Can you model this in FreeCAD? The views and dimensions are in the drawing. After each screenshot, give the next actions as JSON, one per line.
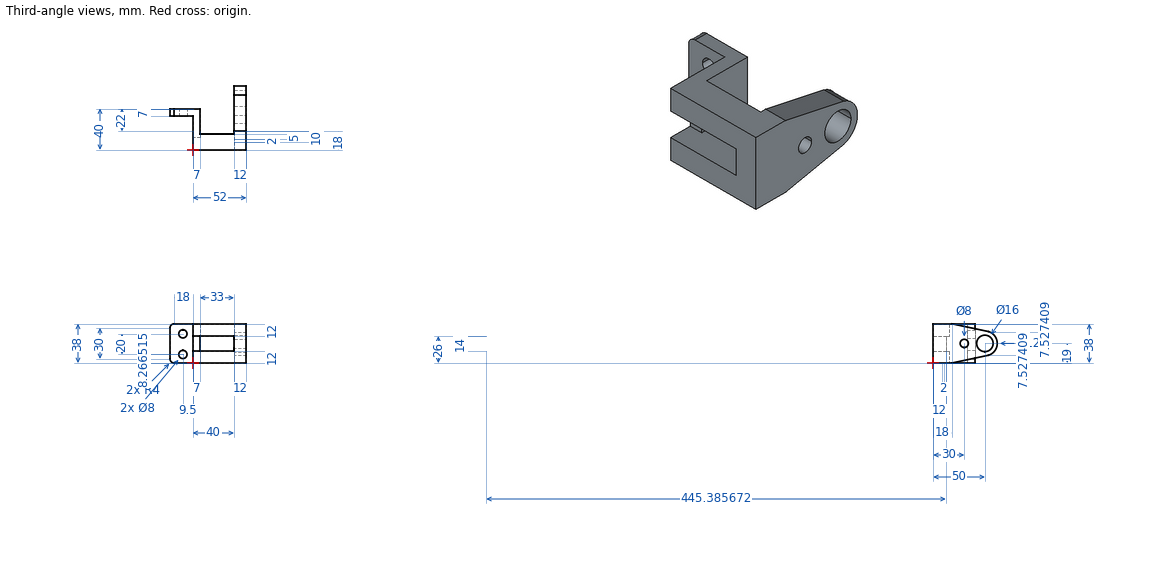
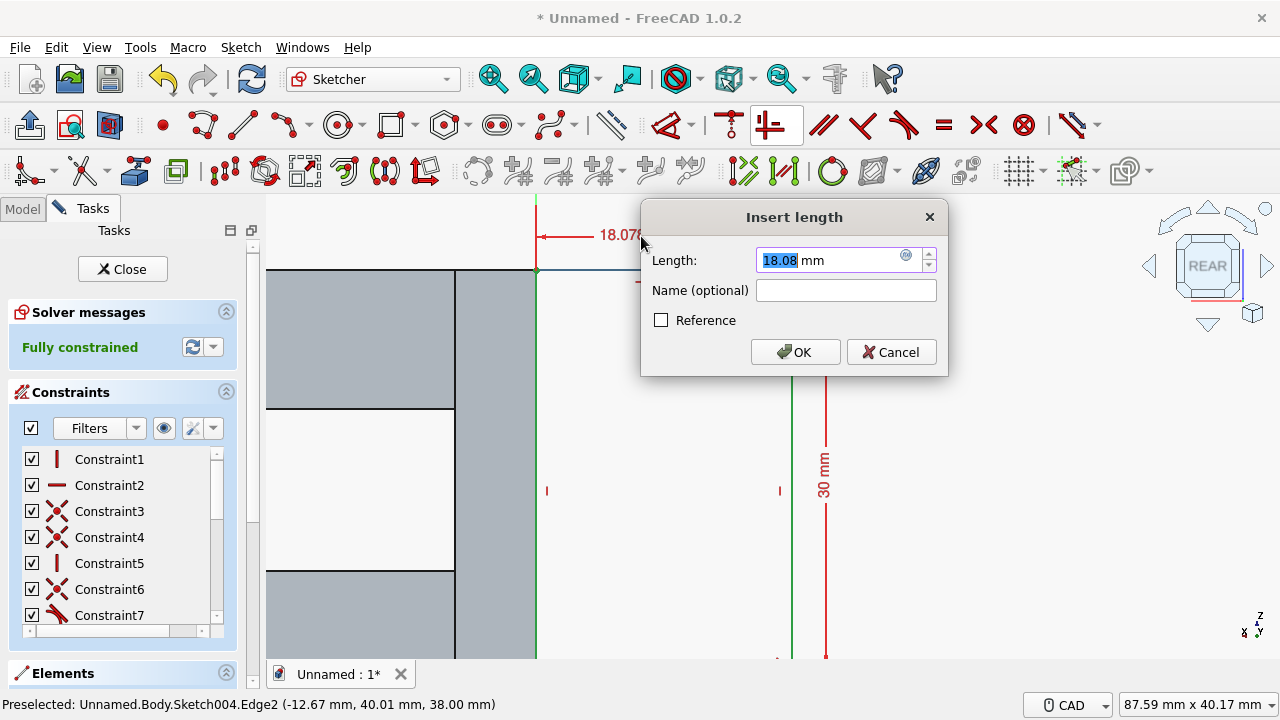
{"action": "type", "text": "18"}
{"action": "key", "text": "Return"}
{"action": "key", "text": "Escape"}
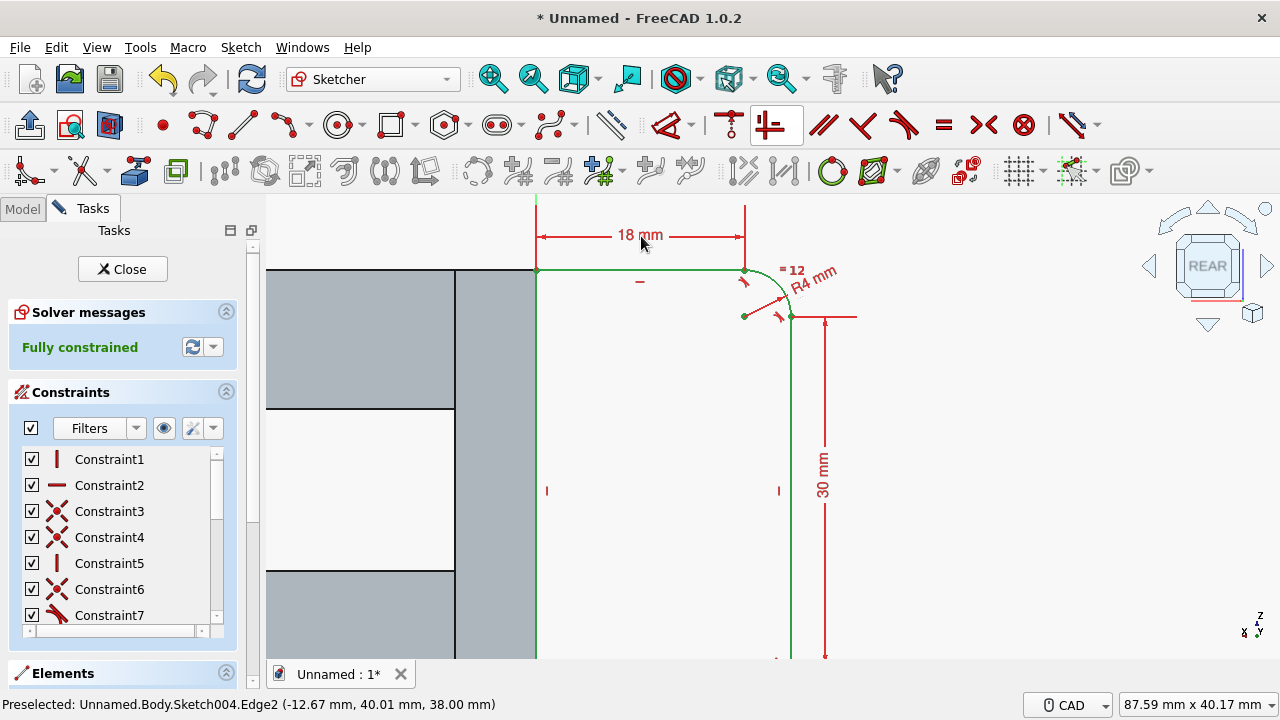
{"action": "left_click", "coordinate": [123, 269]}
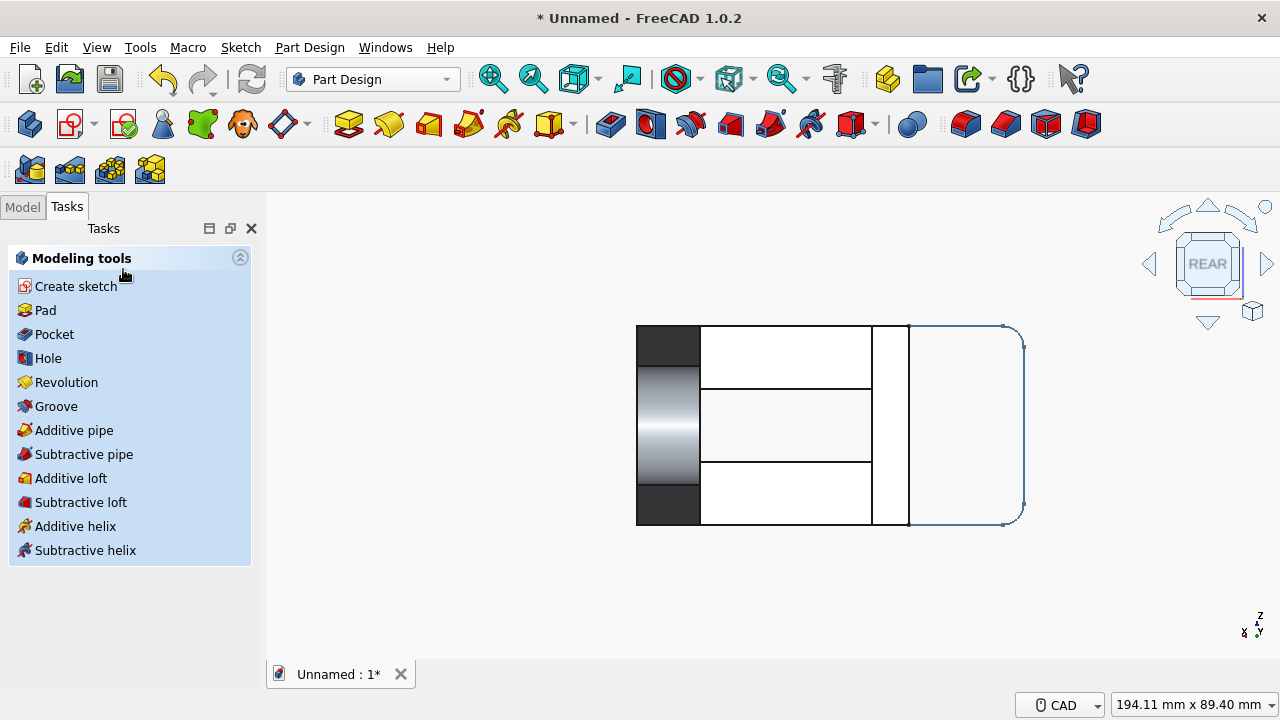
{"action": "left_click", "coordinate": [350, 124]}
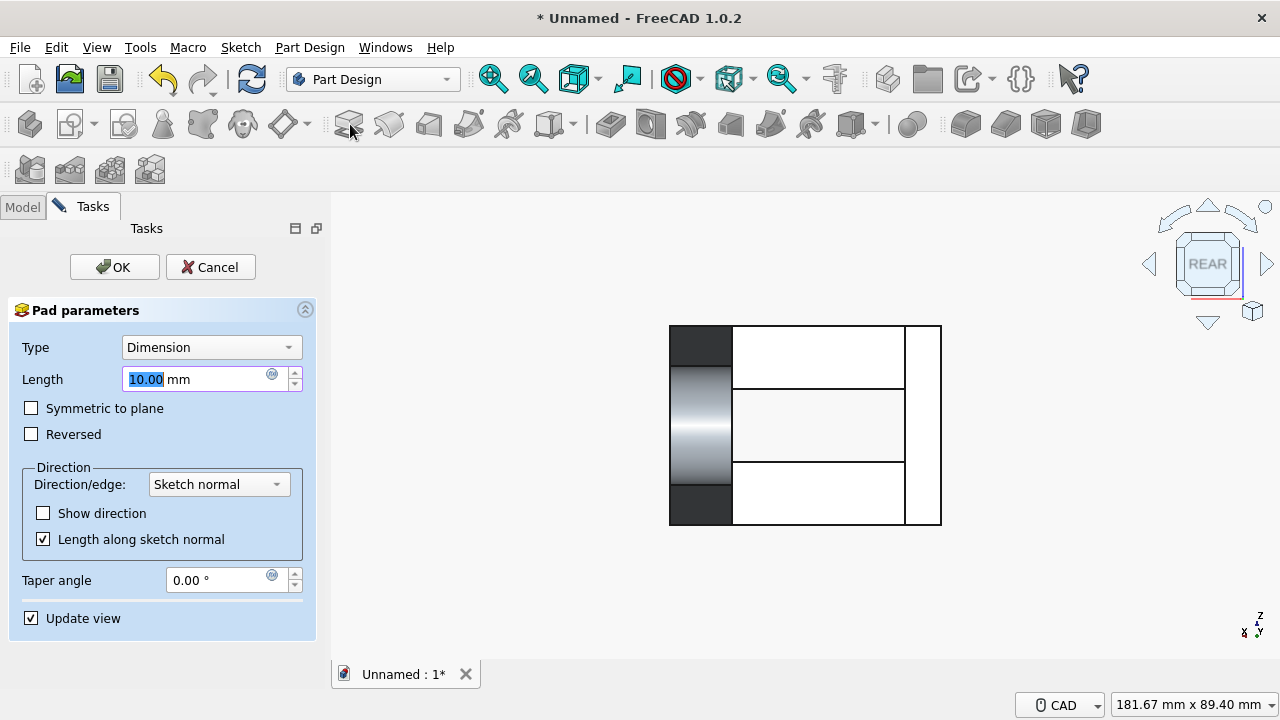
{"action": "type", "text": "7"}
{"action": "key", "text": "Tab"}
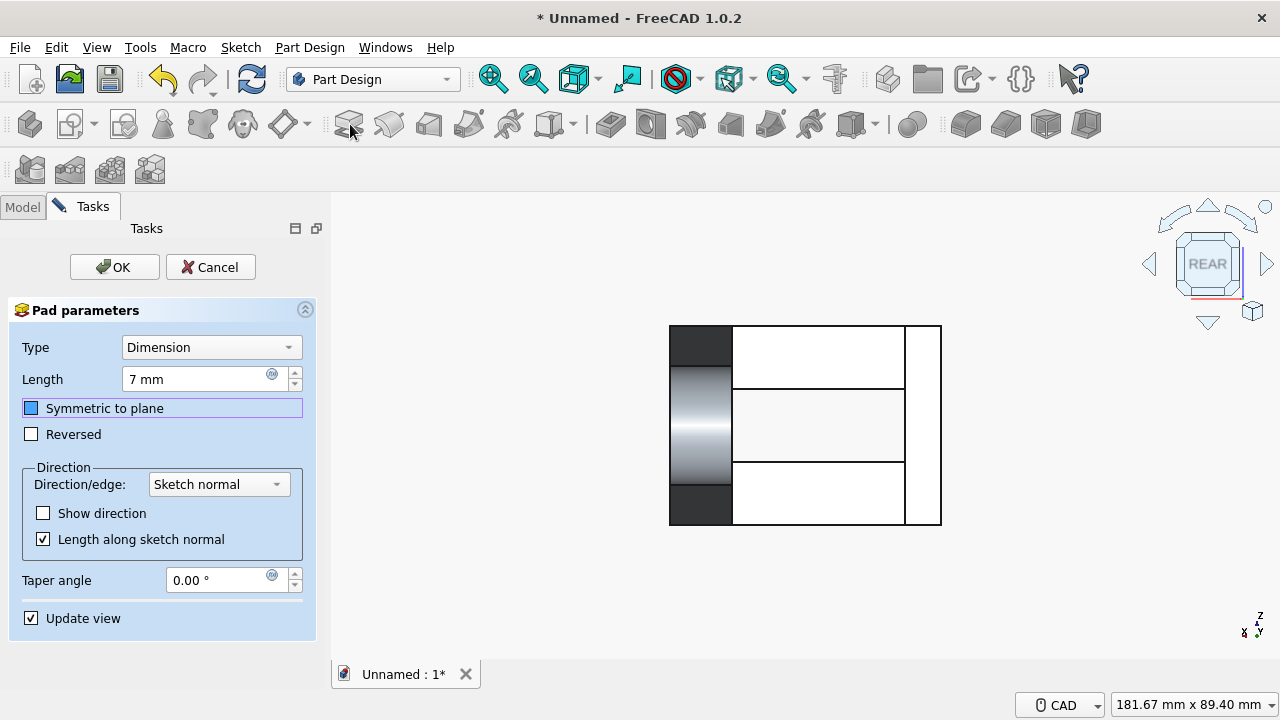
{"action": "left_click", "coordinate": [30, 434]}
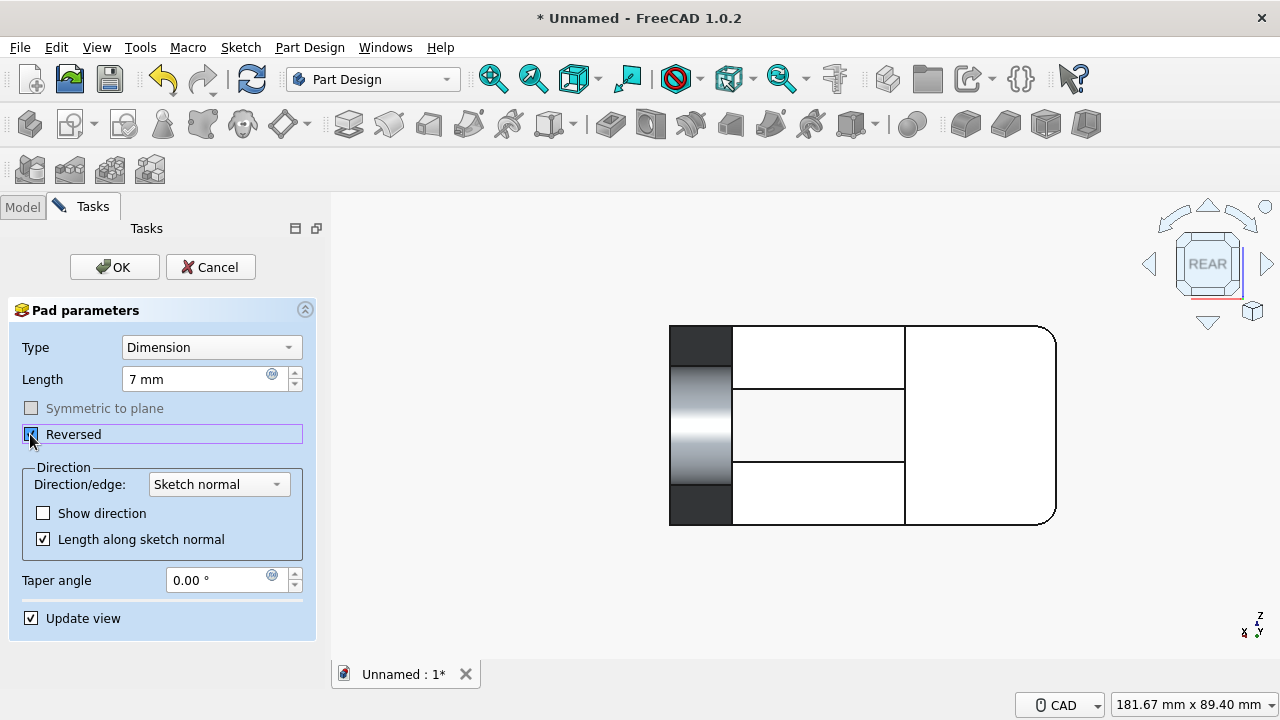
{"action": "left_click", "coordinate": [115, 267]}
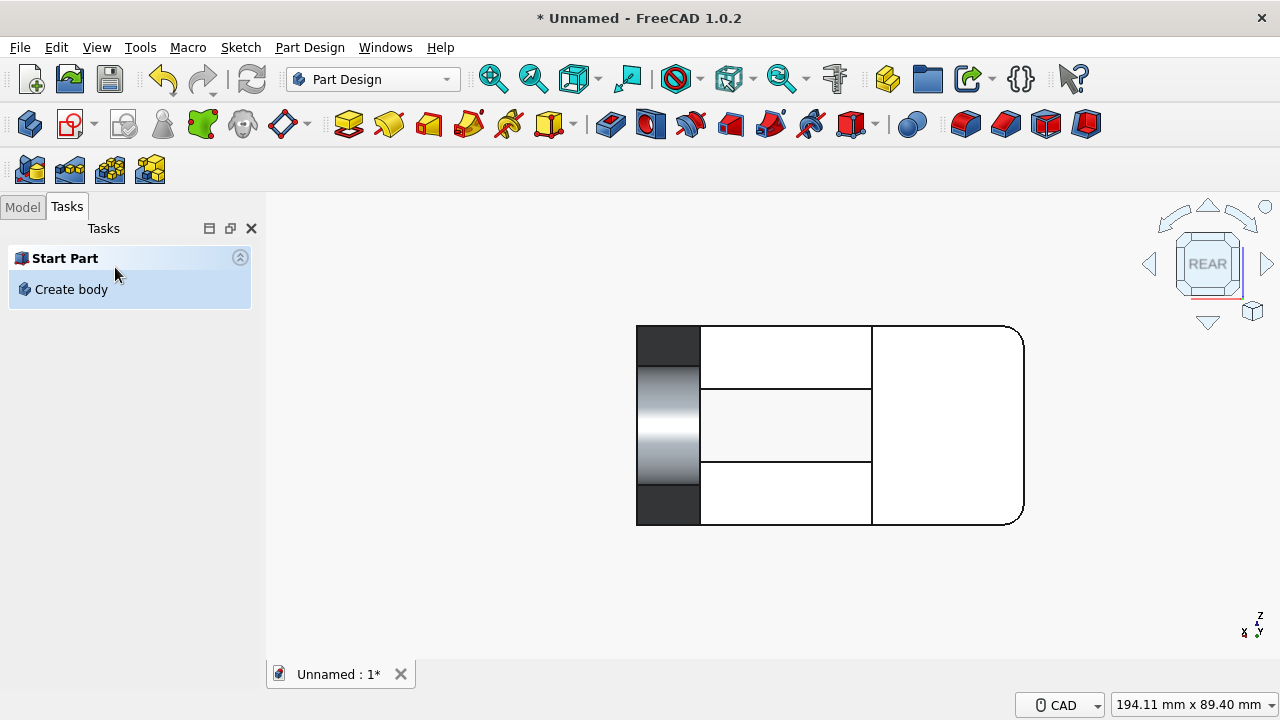
{"action": "left_click", "coordinate": [494, 80]}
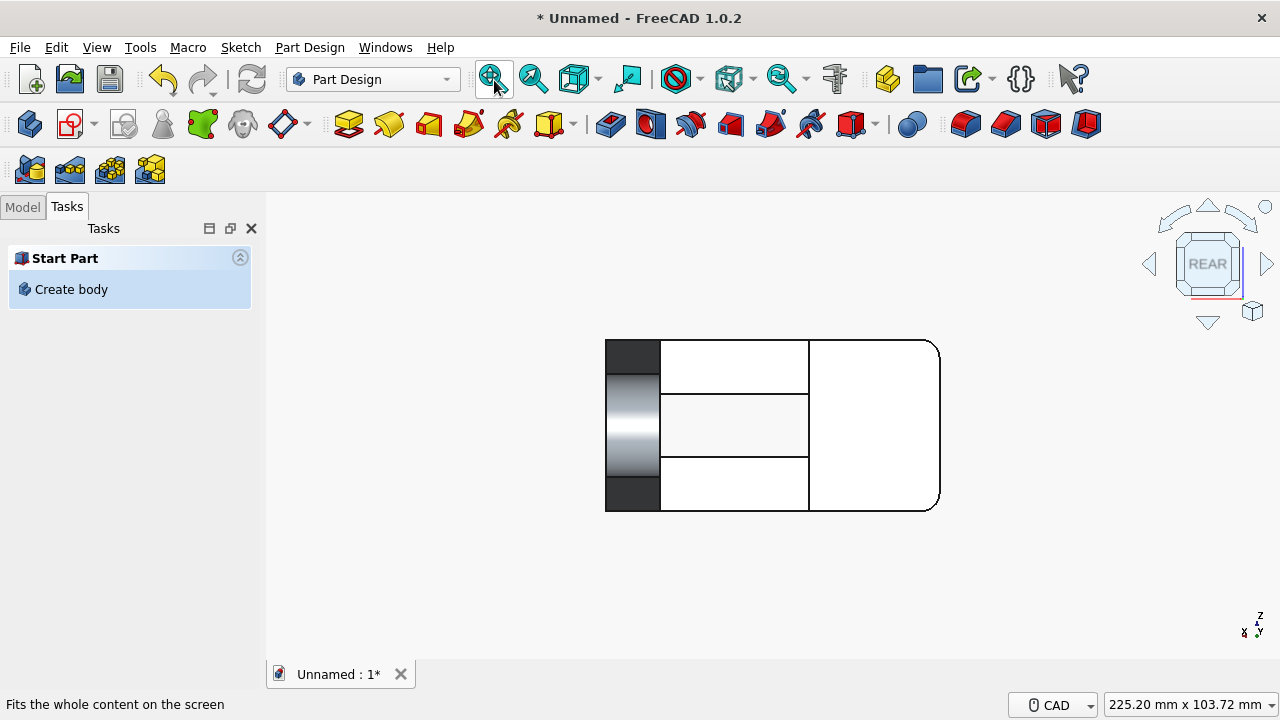
{"action": "left_click", "coordinate": [692, 483]}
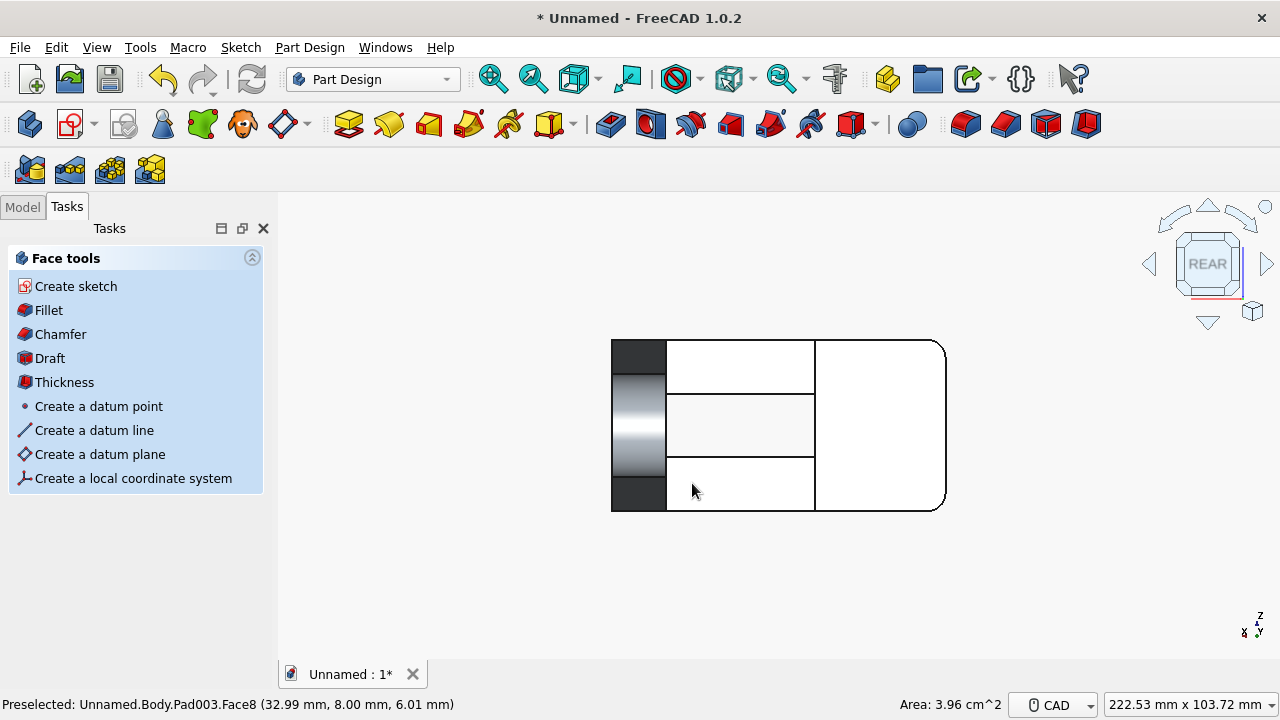
{"action": "left_click", "coordinate": [70, 124]}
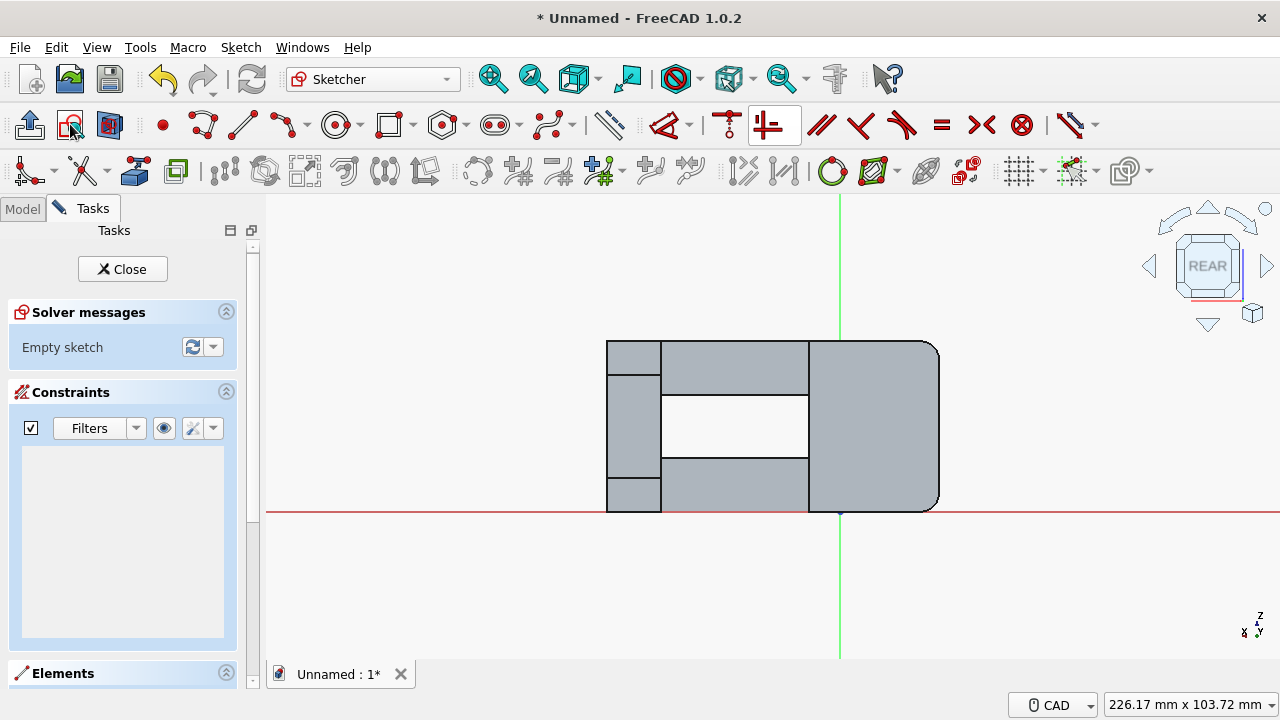
{"action": "left_click", "coordinate": [110, 126]}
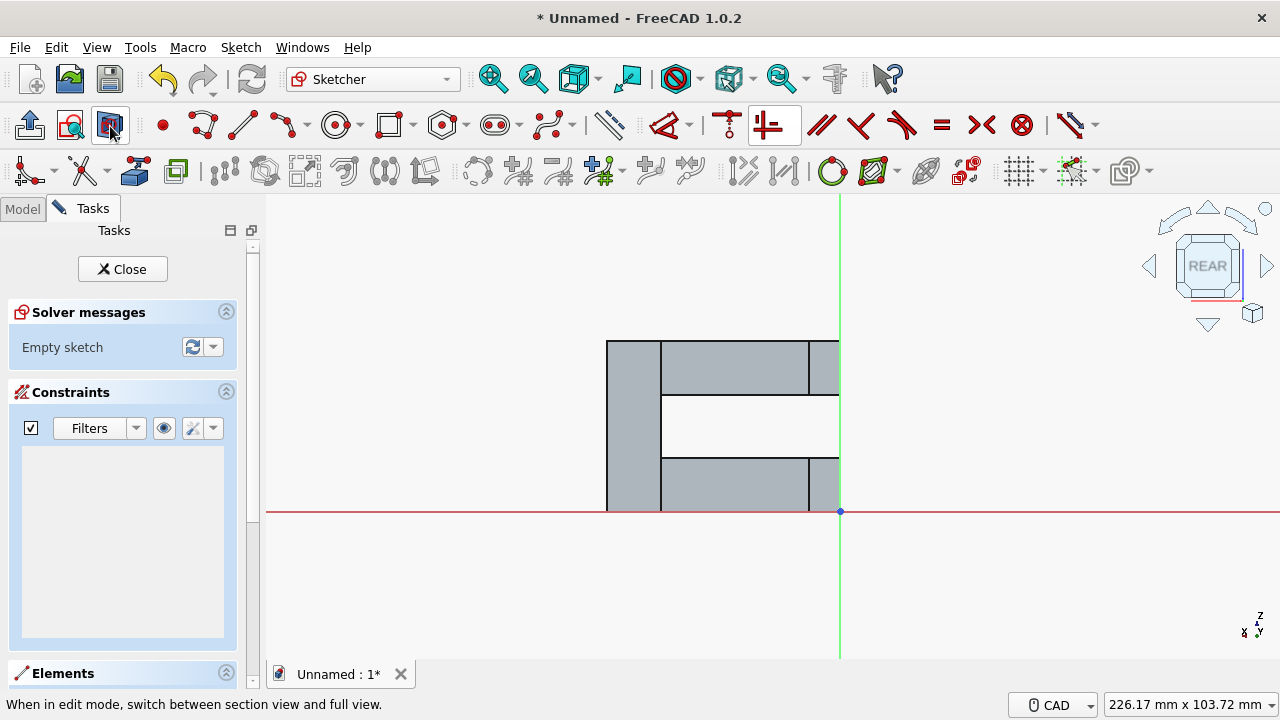
{"action": "scroll", "coordinate": [807, 427], "scroll_direction": "up", "scroll_amount": 3}